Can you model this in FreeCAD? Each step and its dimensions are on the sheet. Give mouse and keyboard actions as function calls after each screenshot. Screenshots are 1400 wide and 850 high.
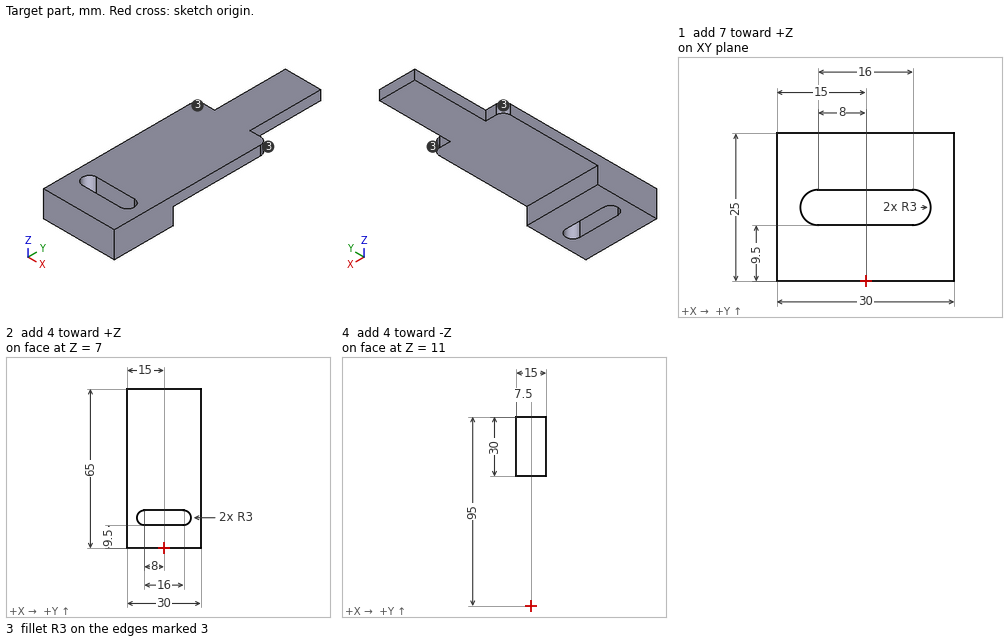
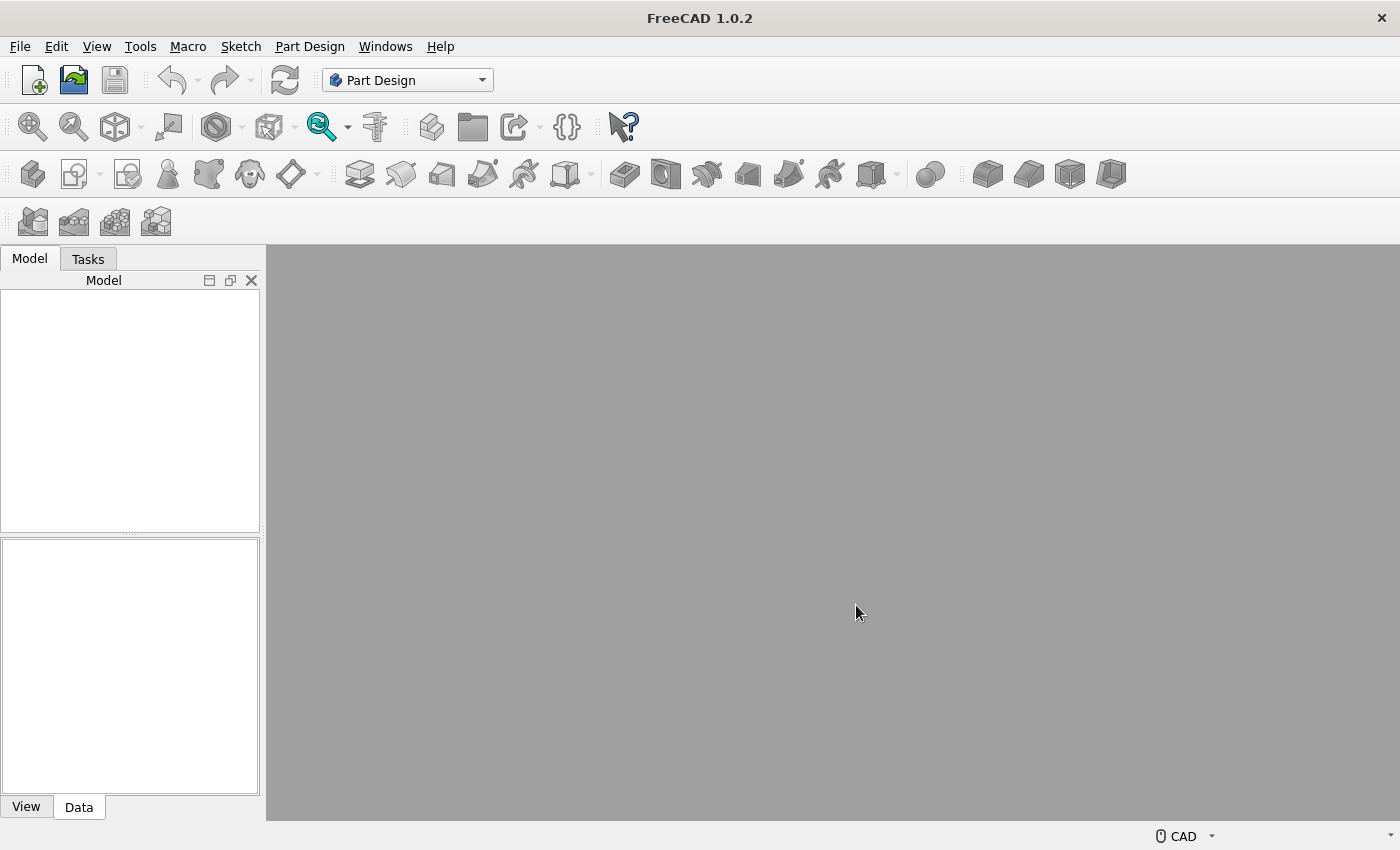
click(33, 80)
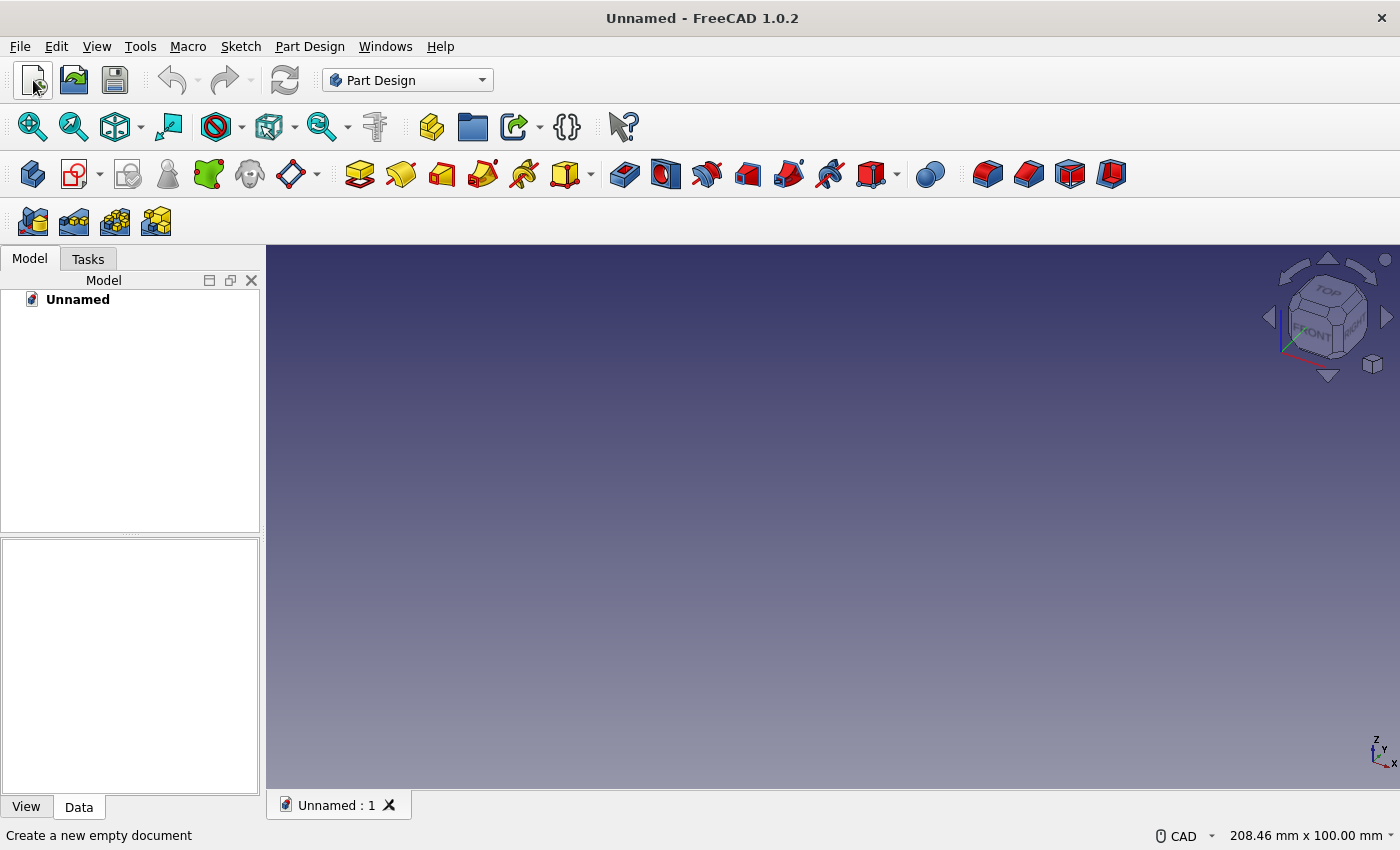
click(74, 174)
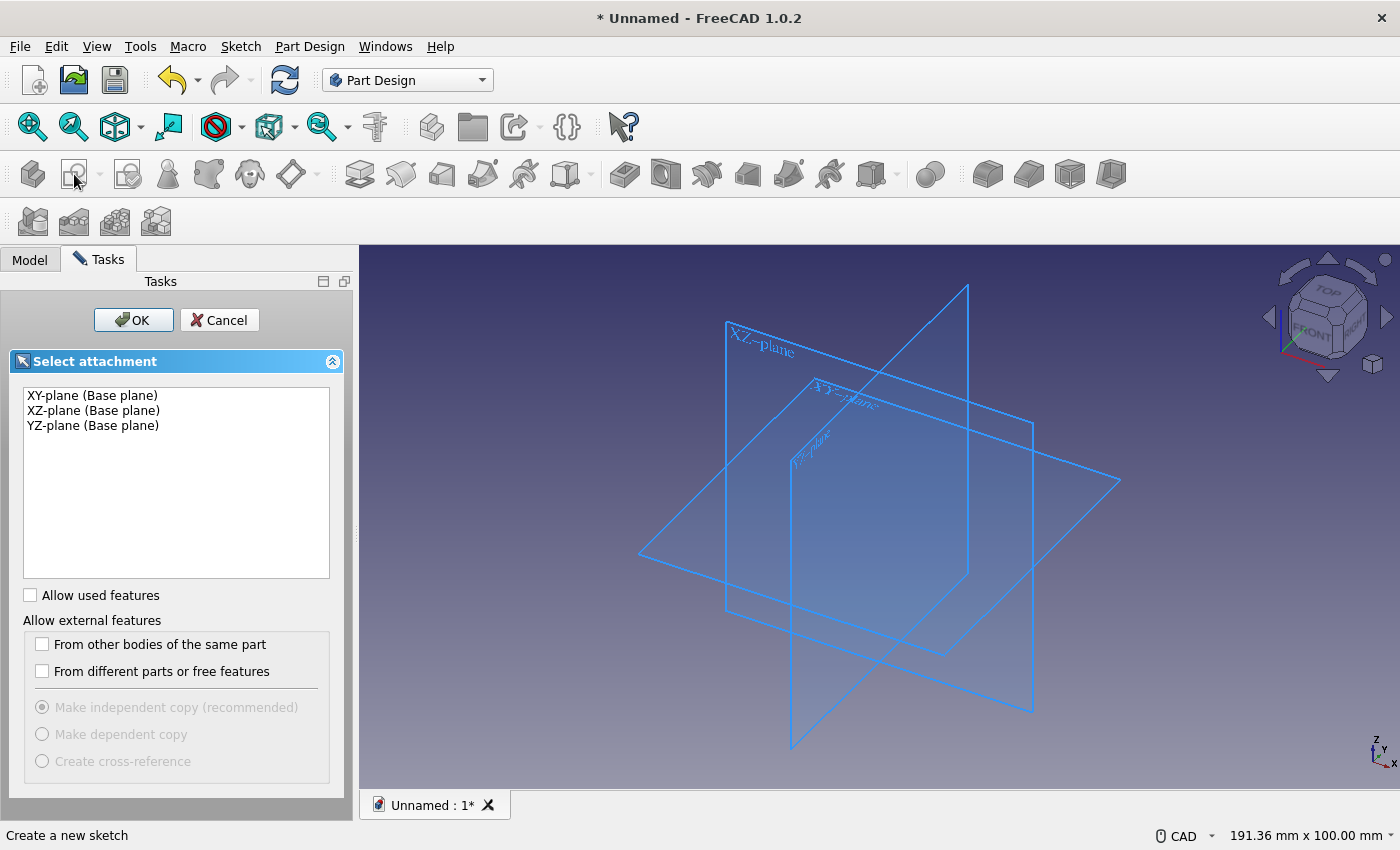
click(84, 396)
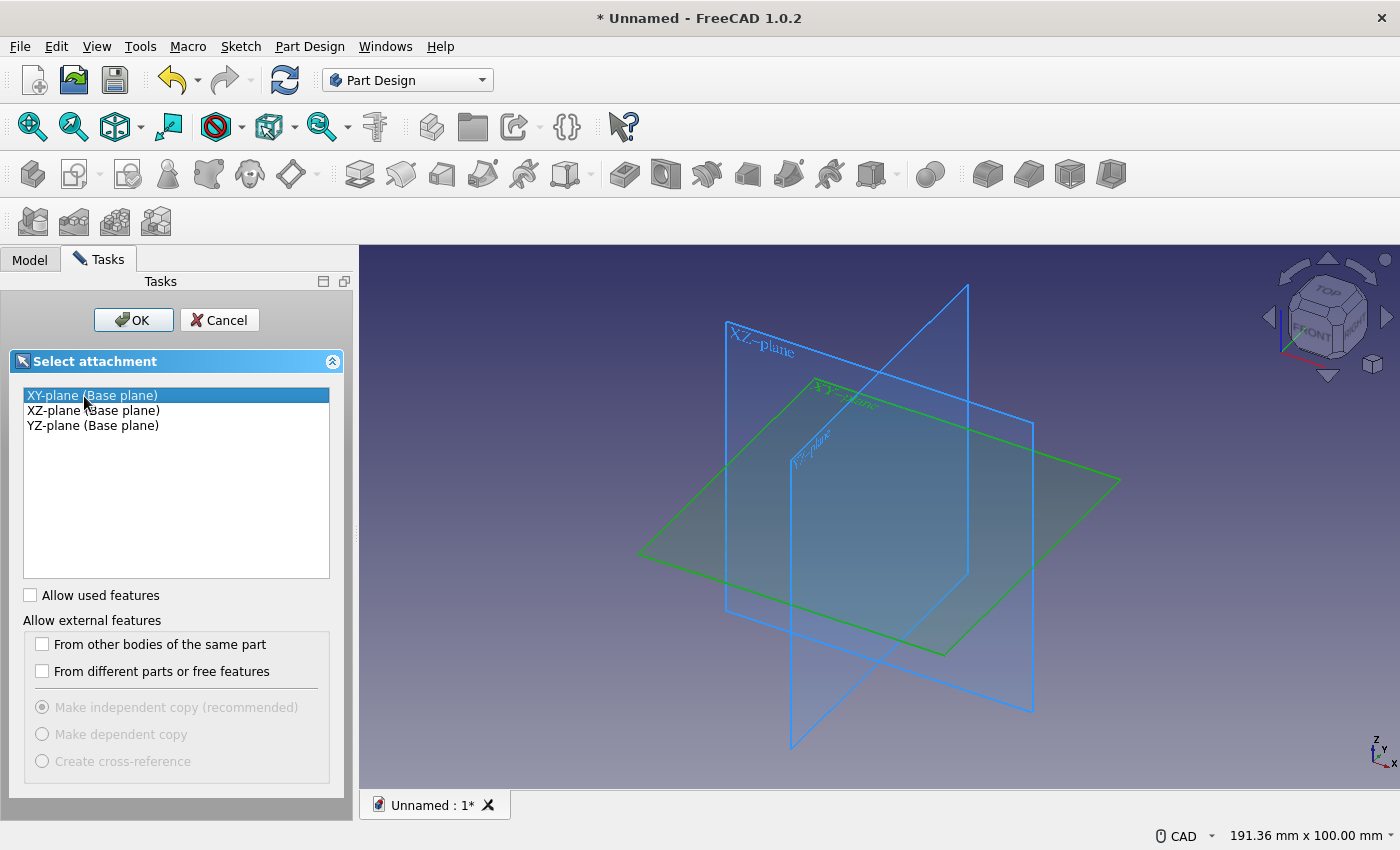
click(134, 320)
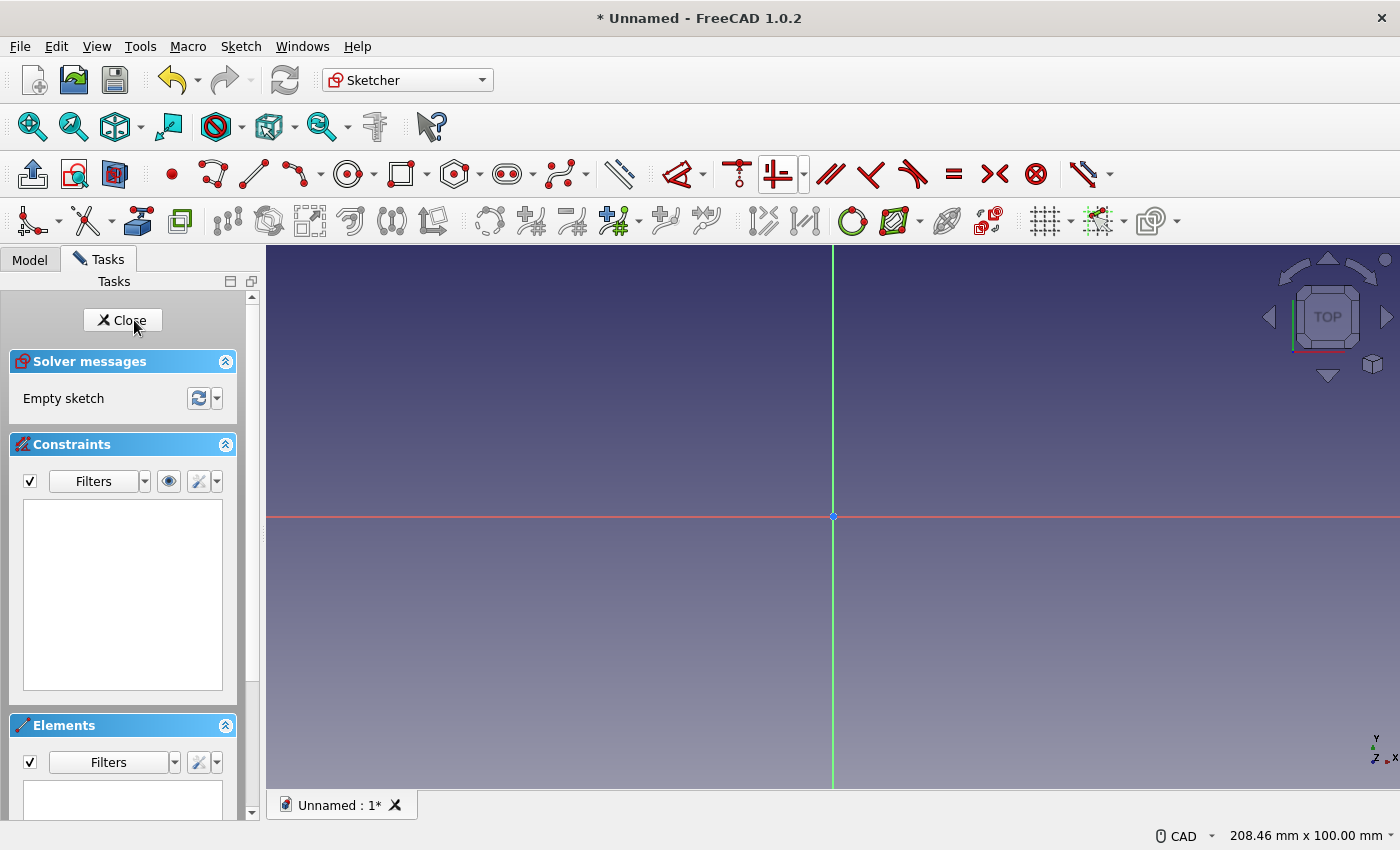
scroll(873, 409, up, 5)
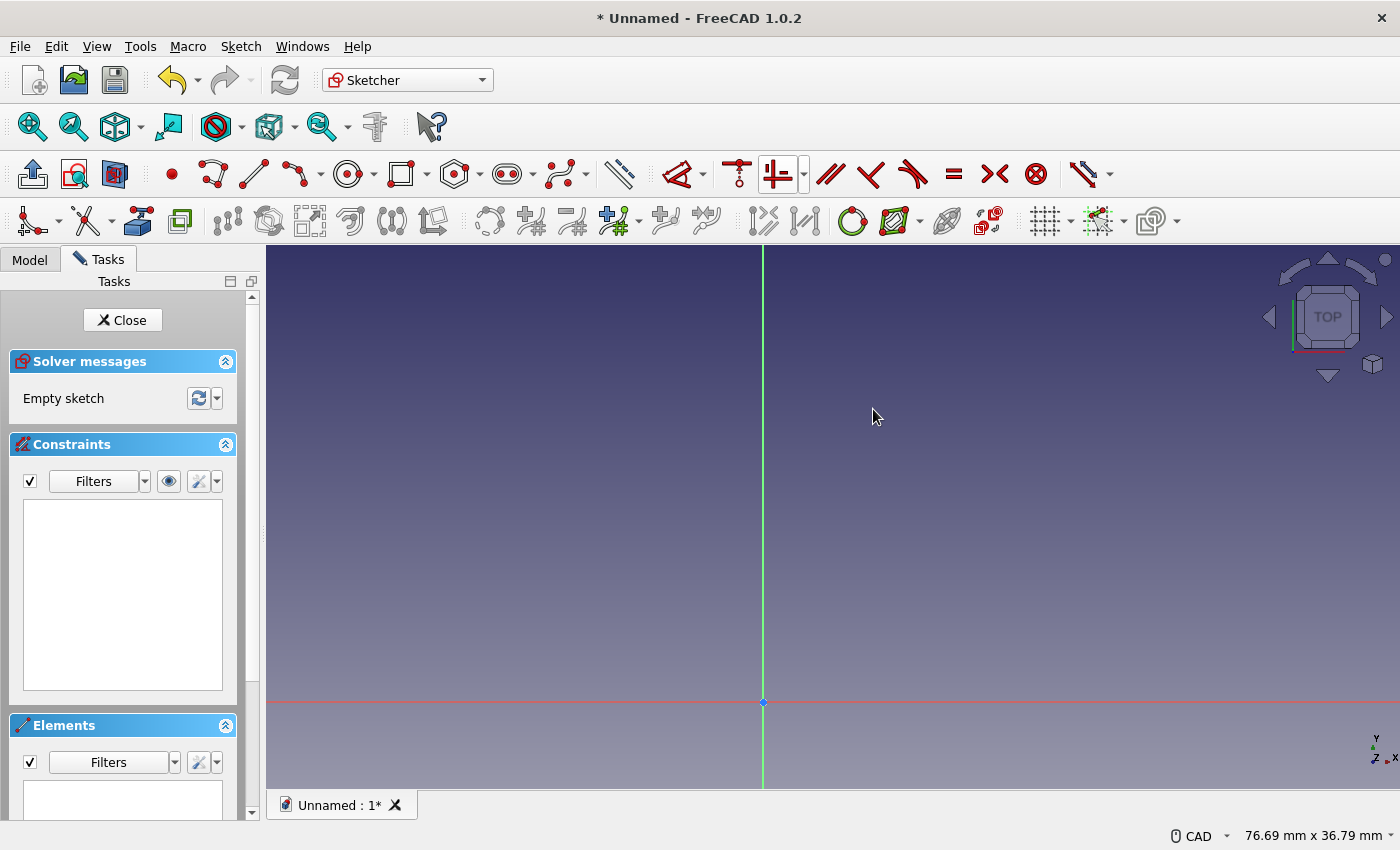
click(400, 174)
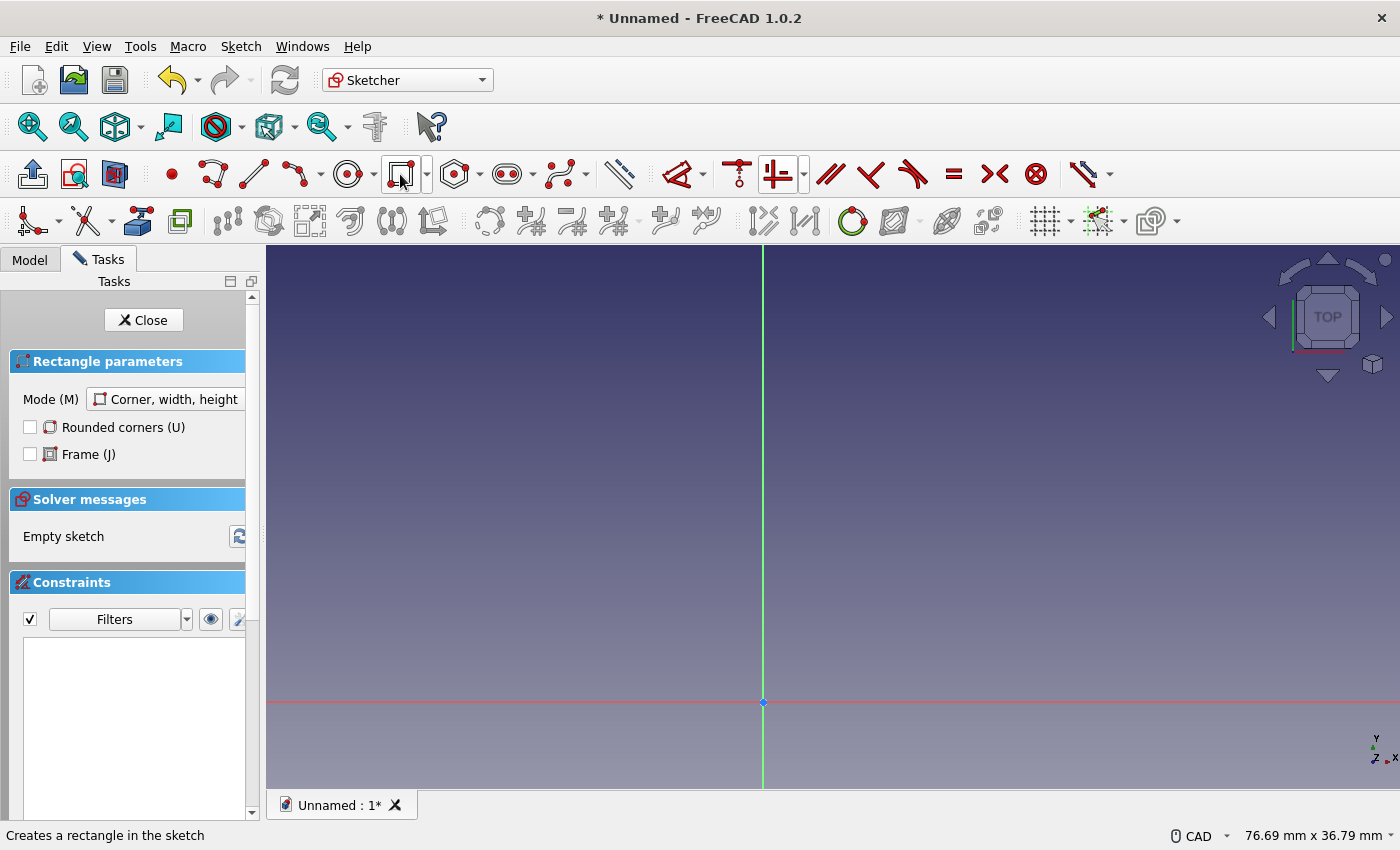
click(542, 332)
click(985, 702)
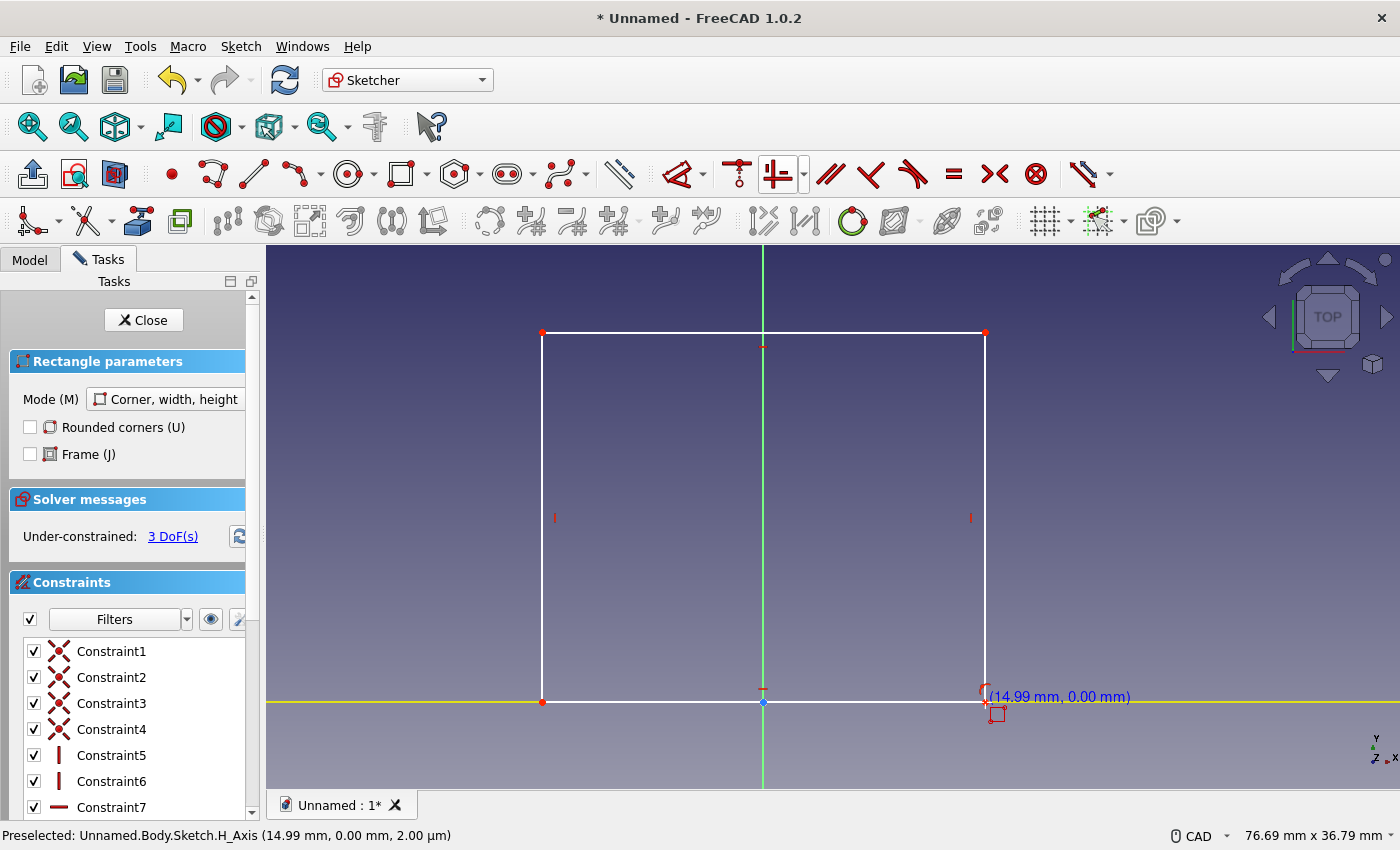
click(506, 174)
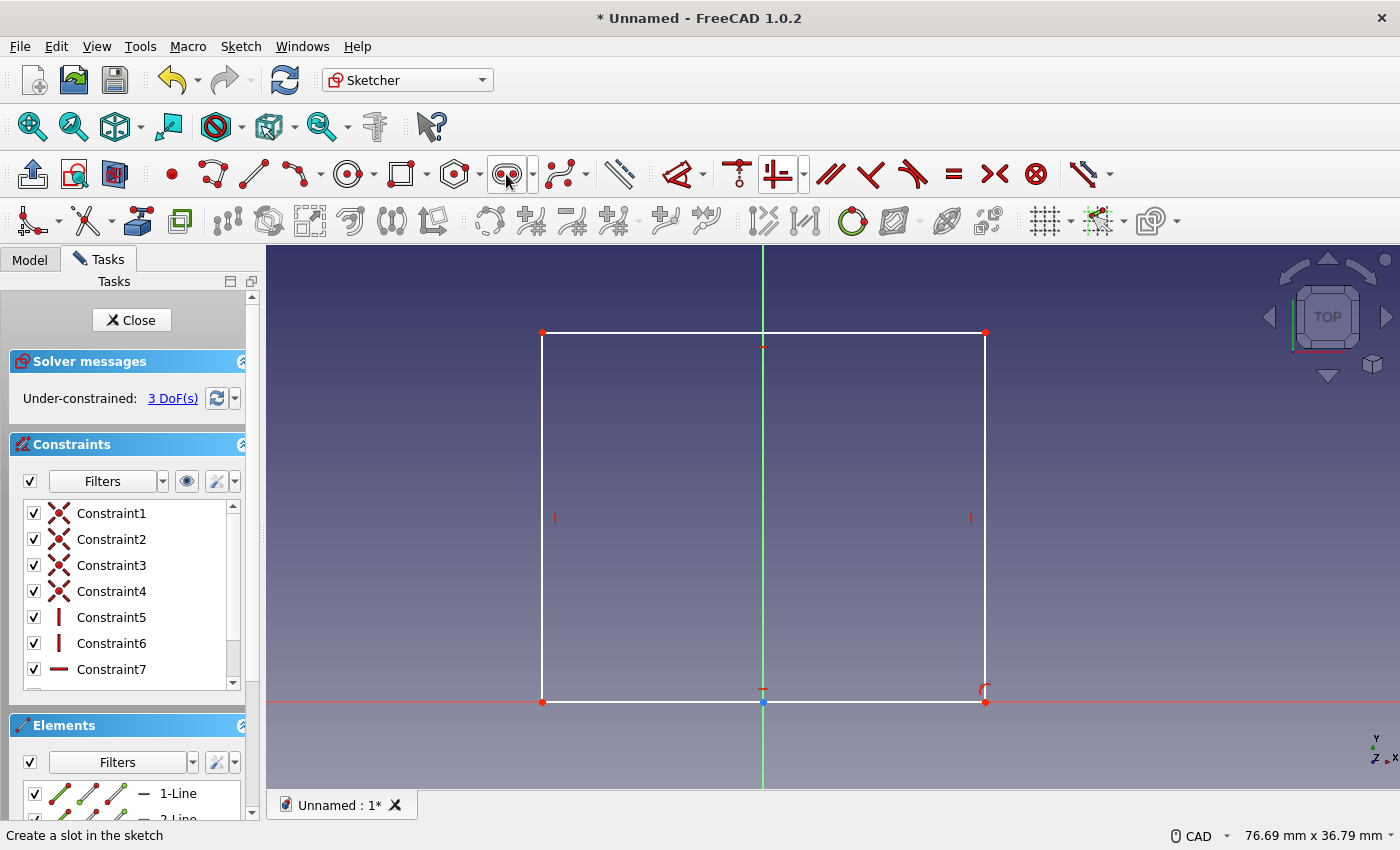
click(645, 517)